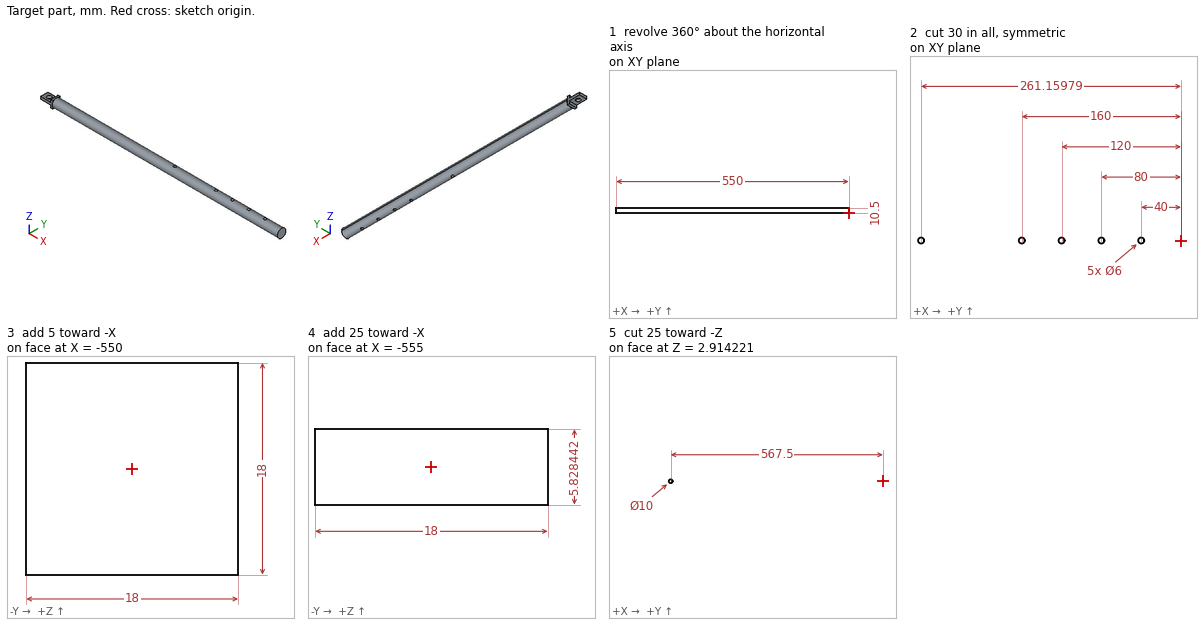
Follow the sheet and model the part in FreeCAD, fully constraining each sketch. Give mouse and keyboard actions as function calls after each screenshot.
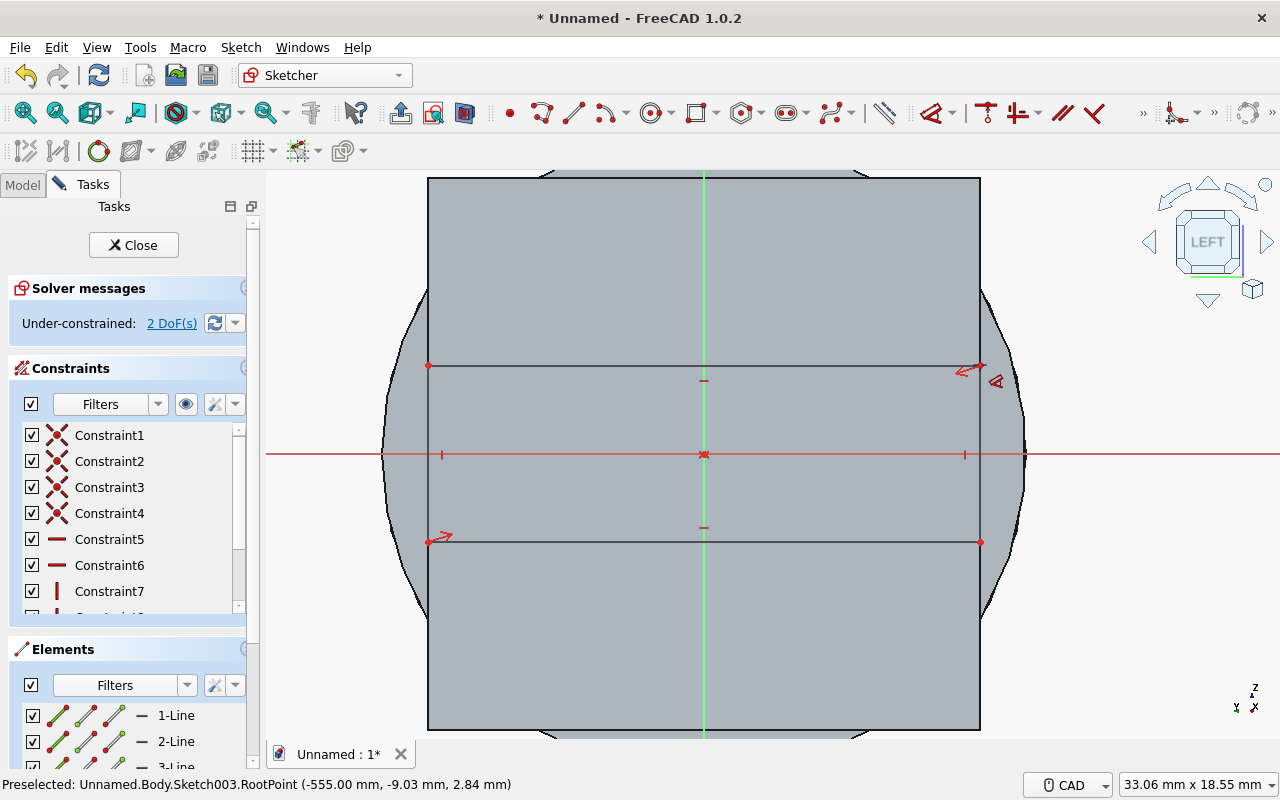
click(594, 542)
click(577, 576)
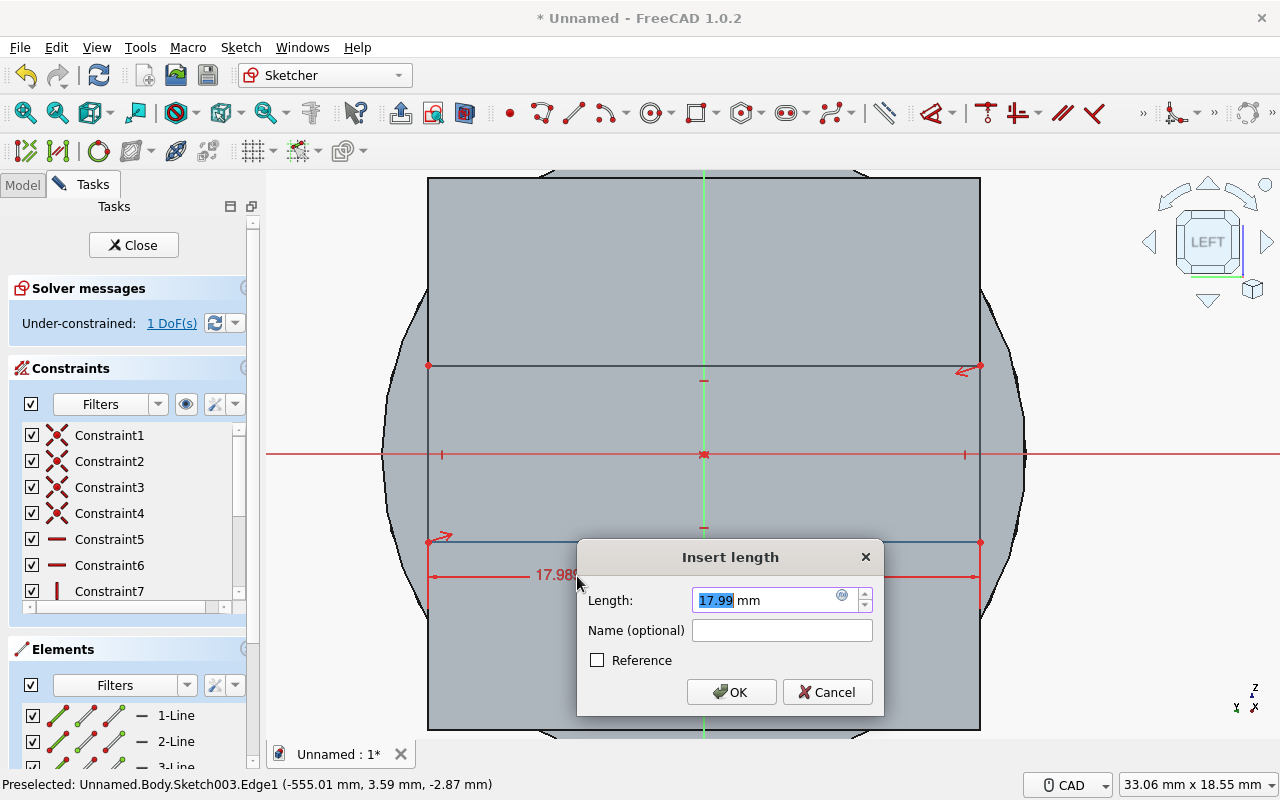
text(18)
key(Return)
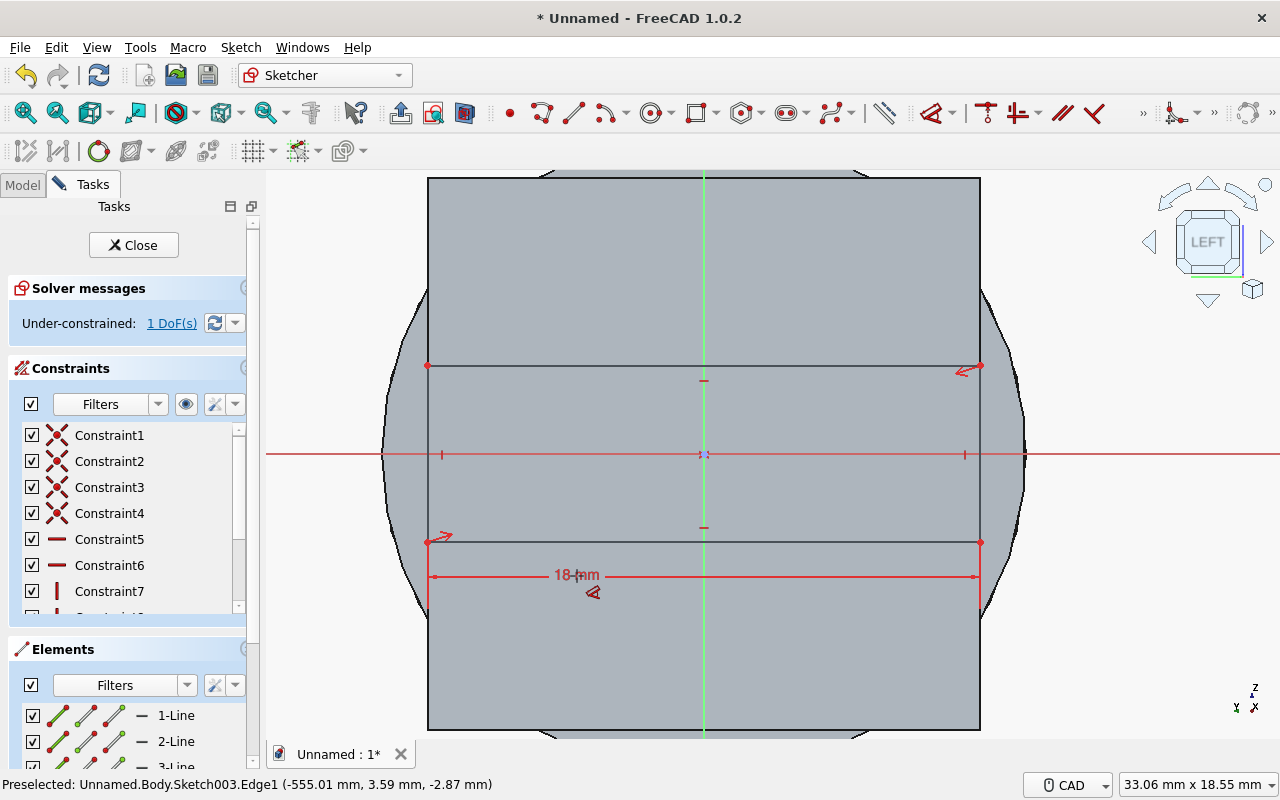
click(980, 489)
click(1014, 414)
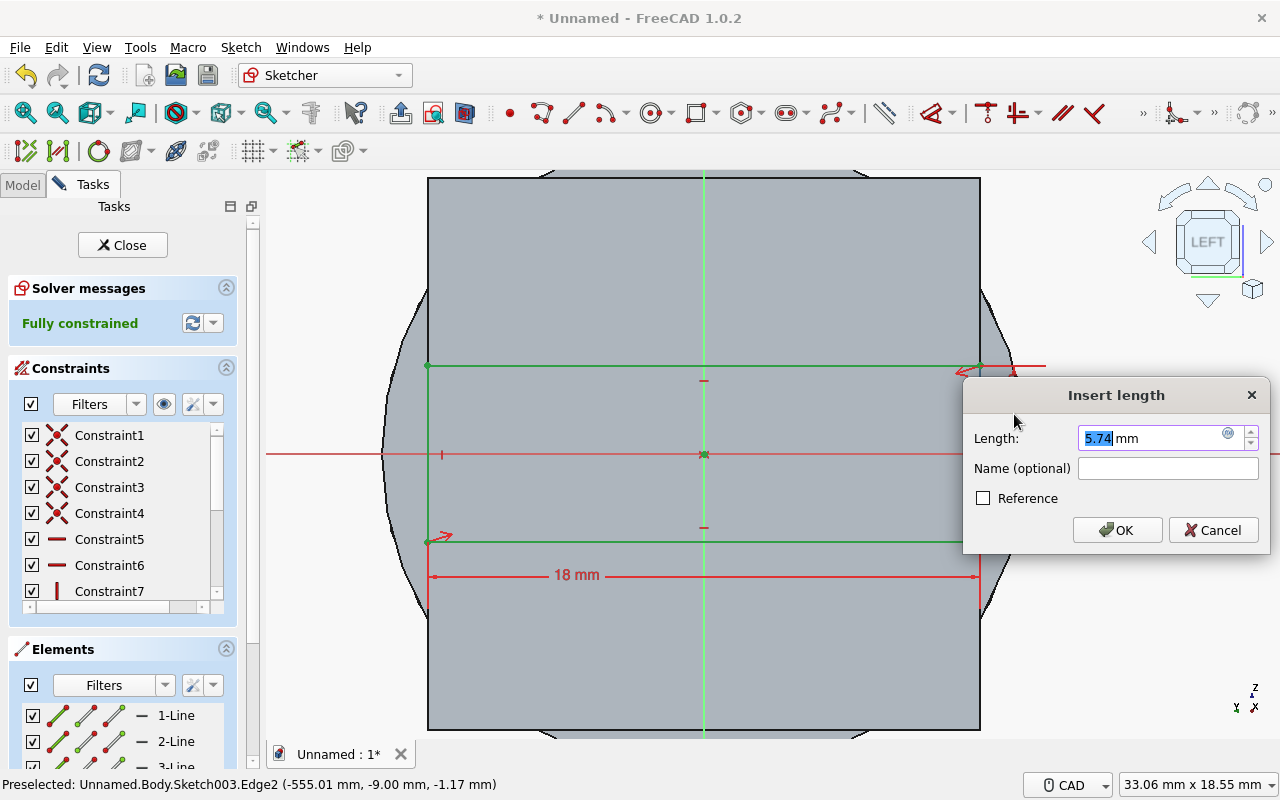
text(5.828442)
key(Return)
key(Escape)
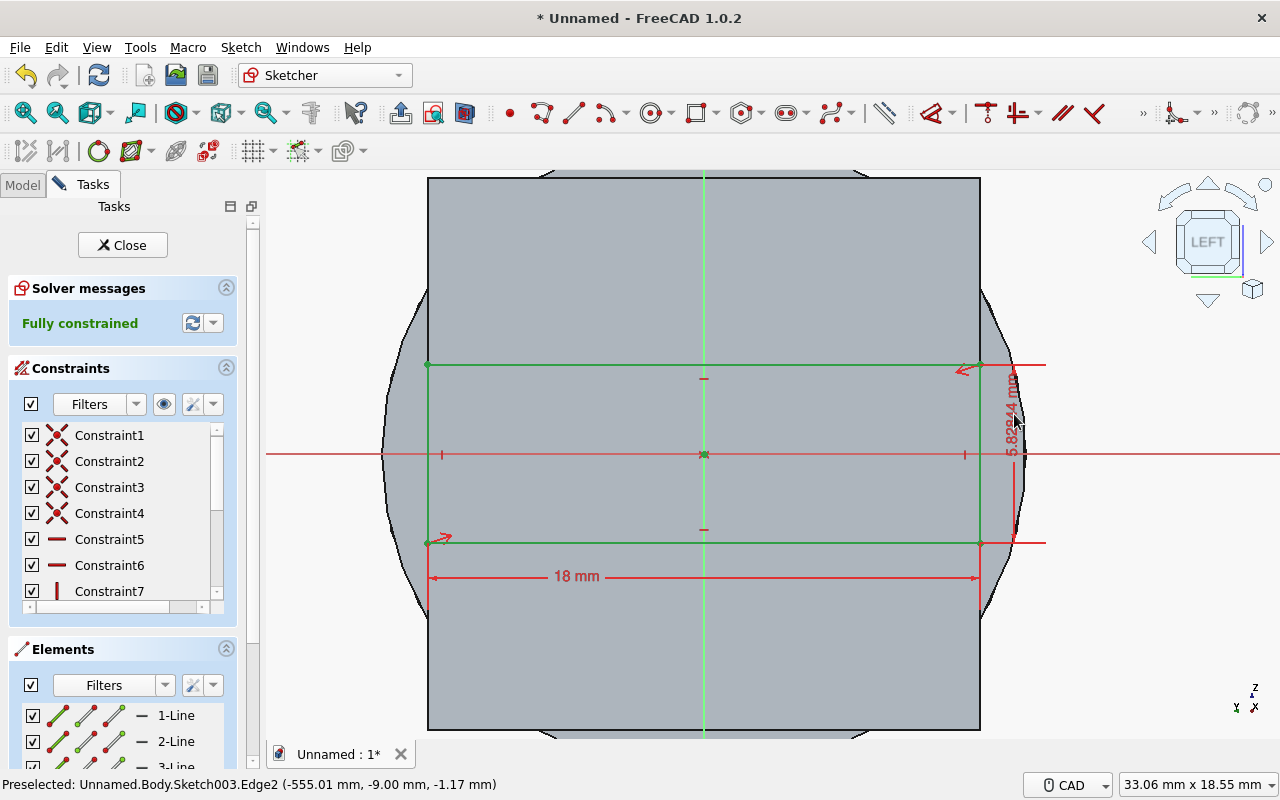
click(123, 245)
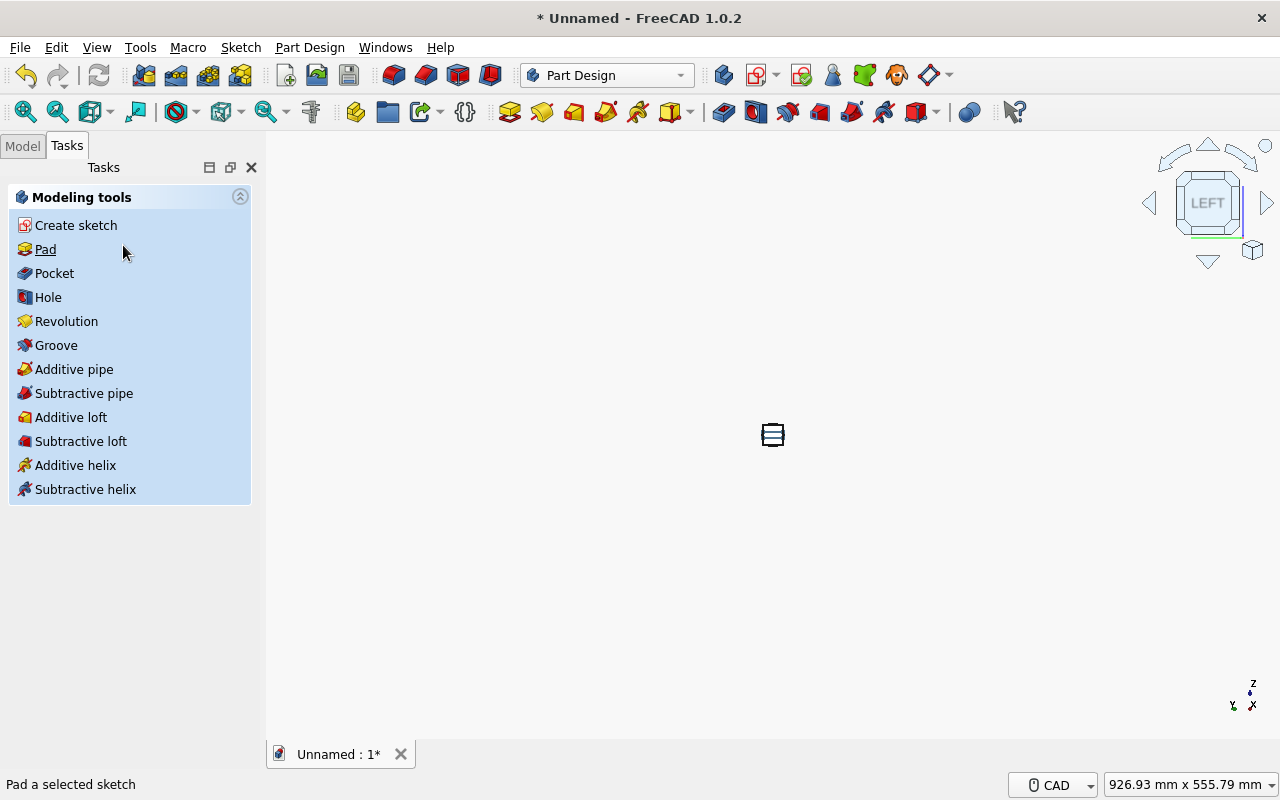
click(510, 112)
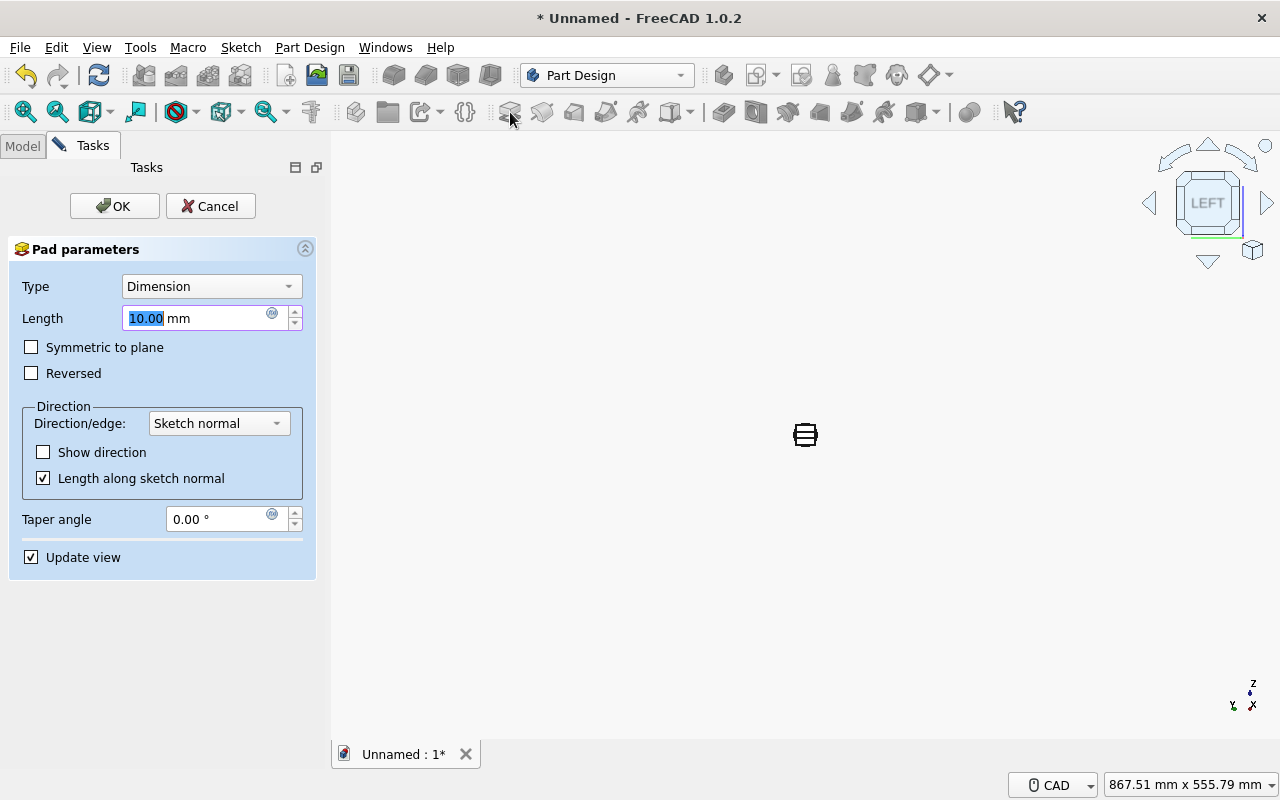
text(25)
key(Tab)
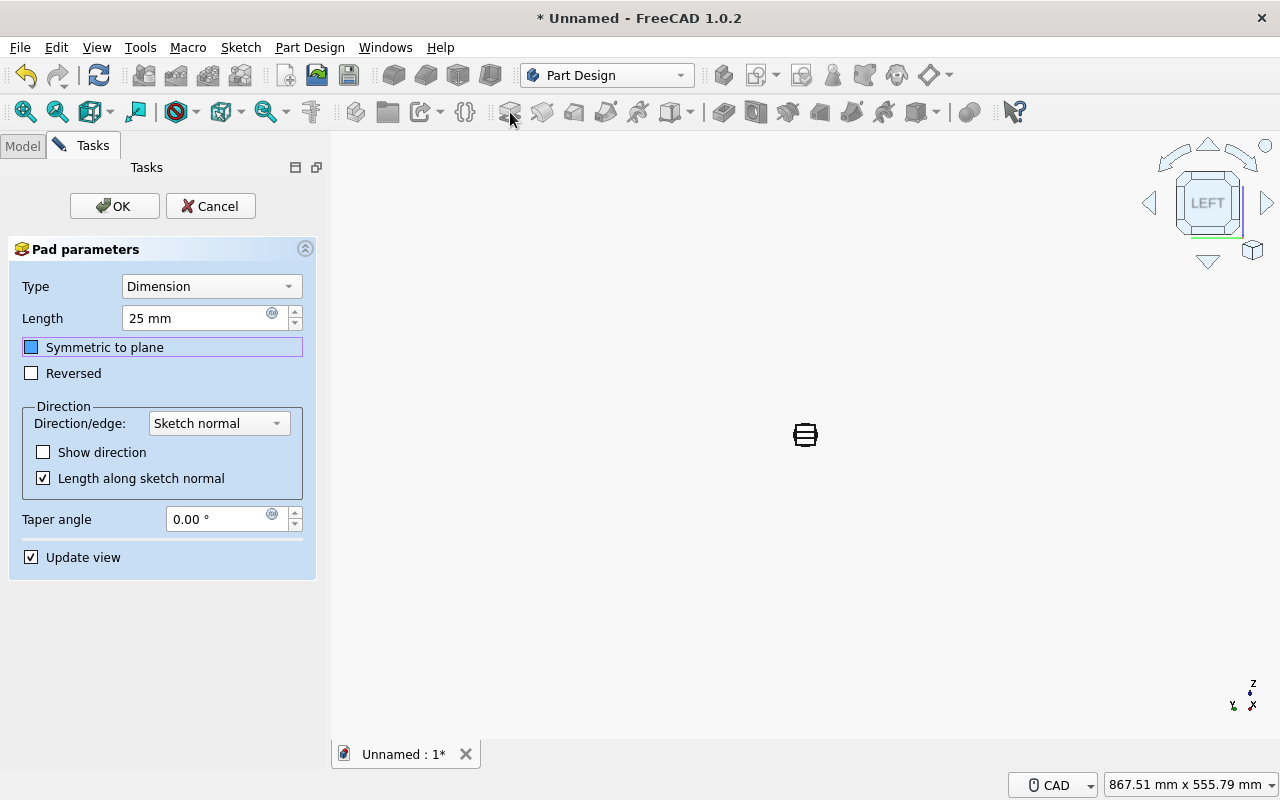
click(115, 206)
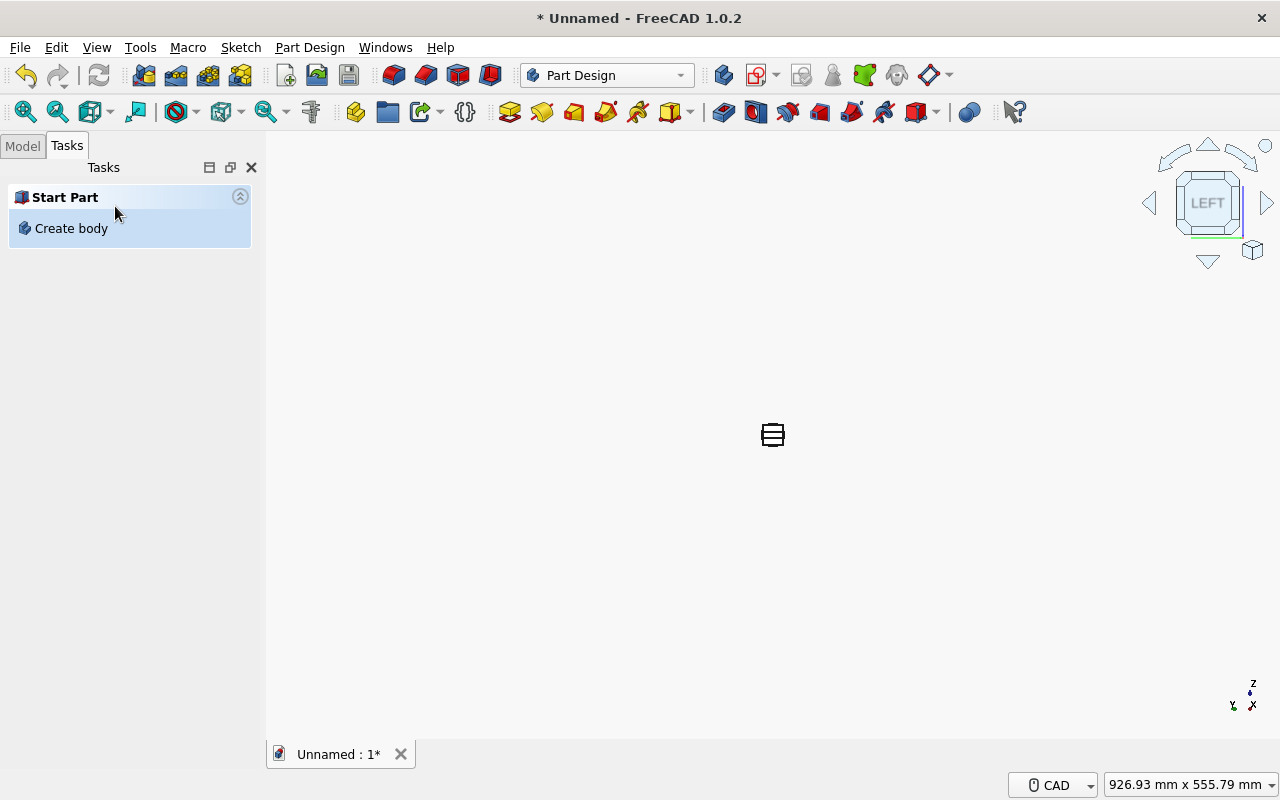
key(v)
key(f)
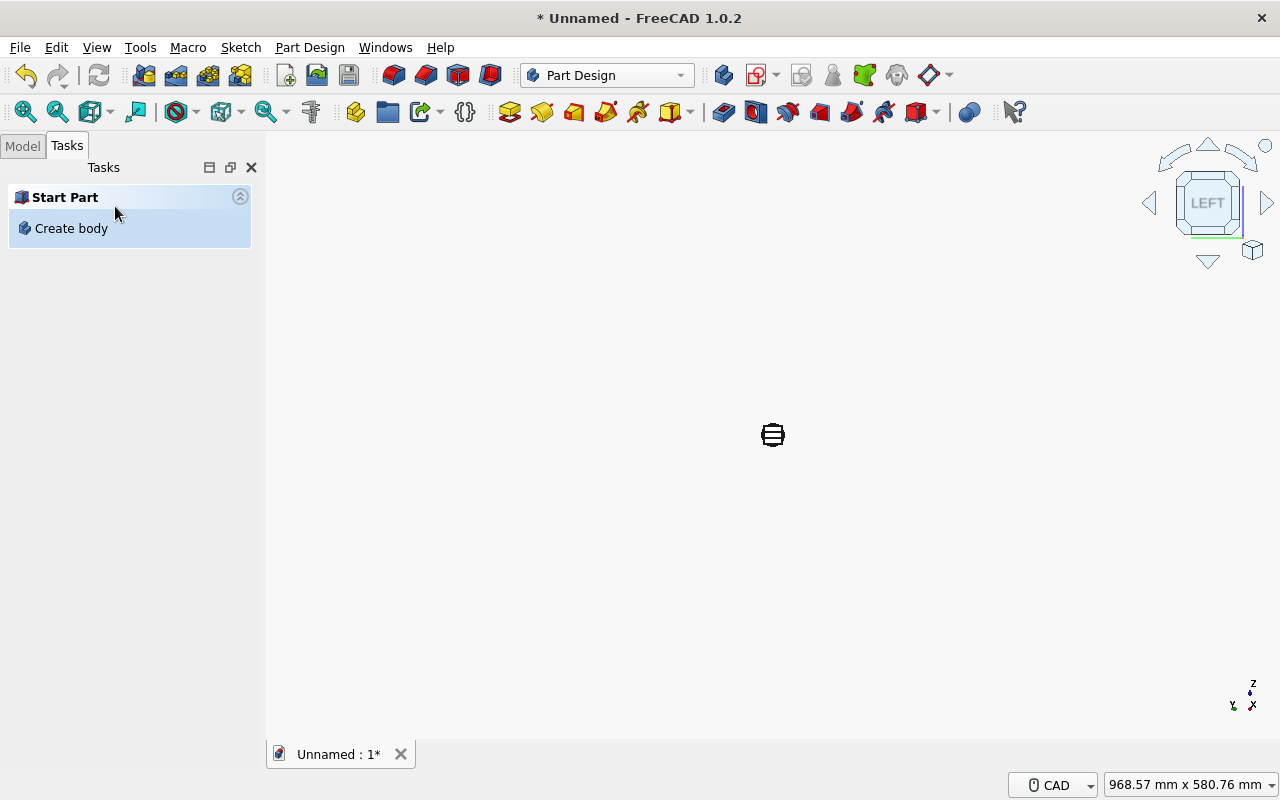
key(0)